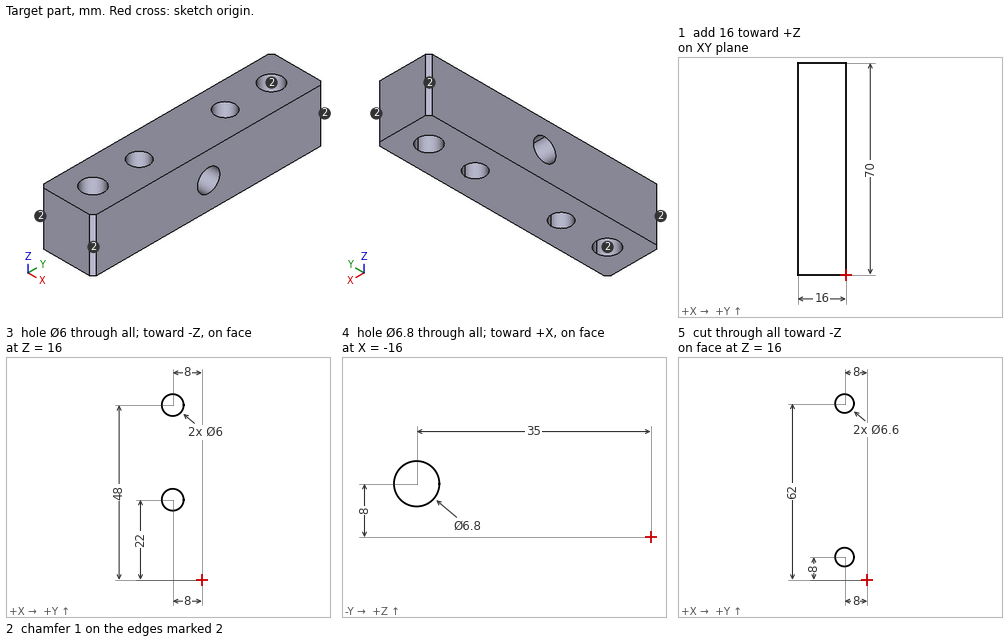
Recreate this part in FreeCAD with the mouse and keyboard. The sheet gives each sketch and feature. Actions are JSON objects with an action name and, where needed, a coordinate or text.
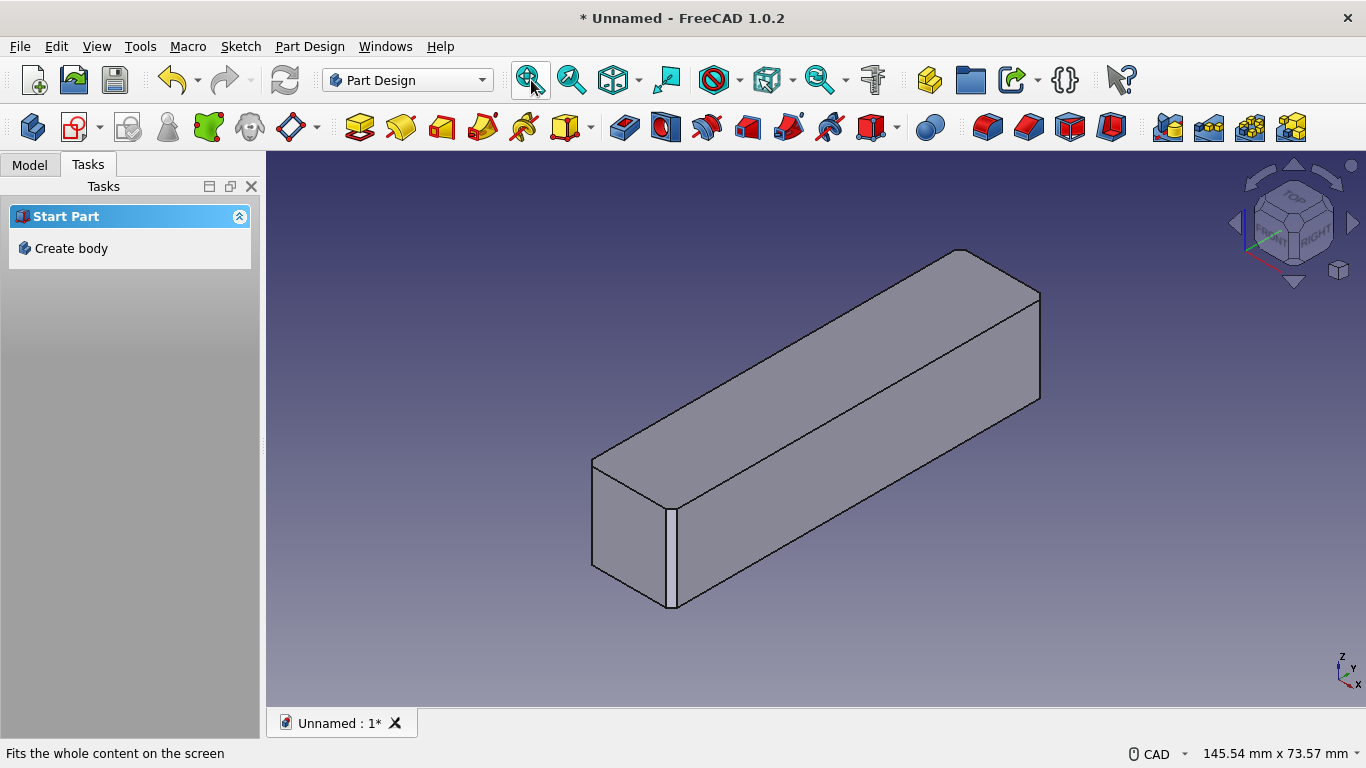
{"action": "left_click", "coordinate": [923, 317]}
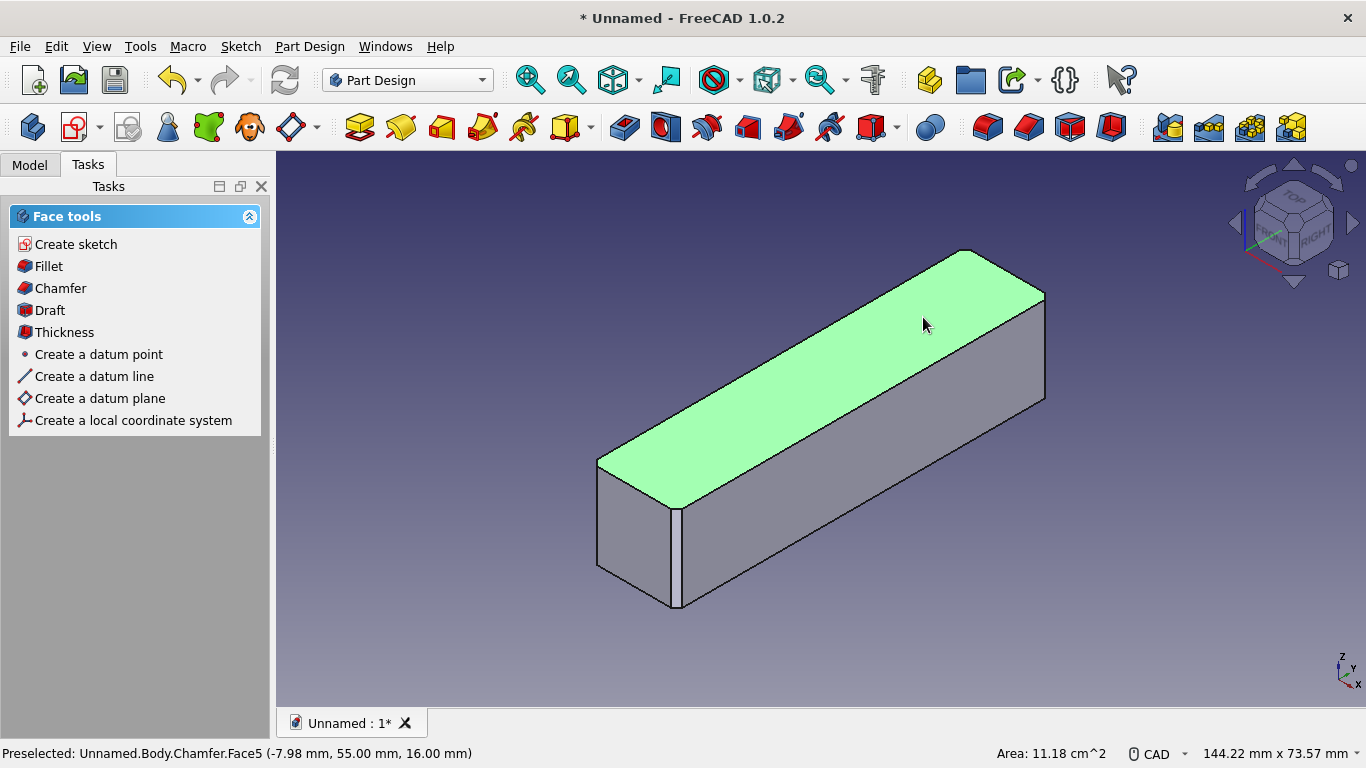
{"action": "left_click", "coordinate": [74, 128]}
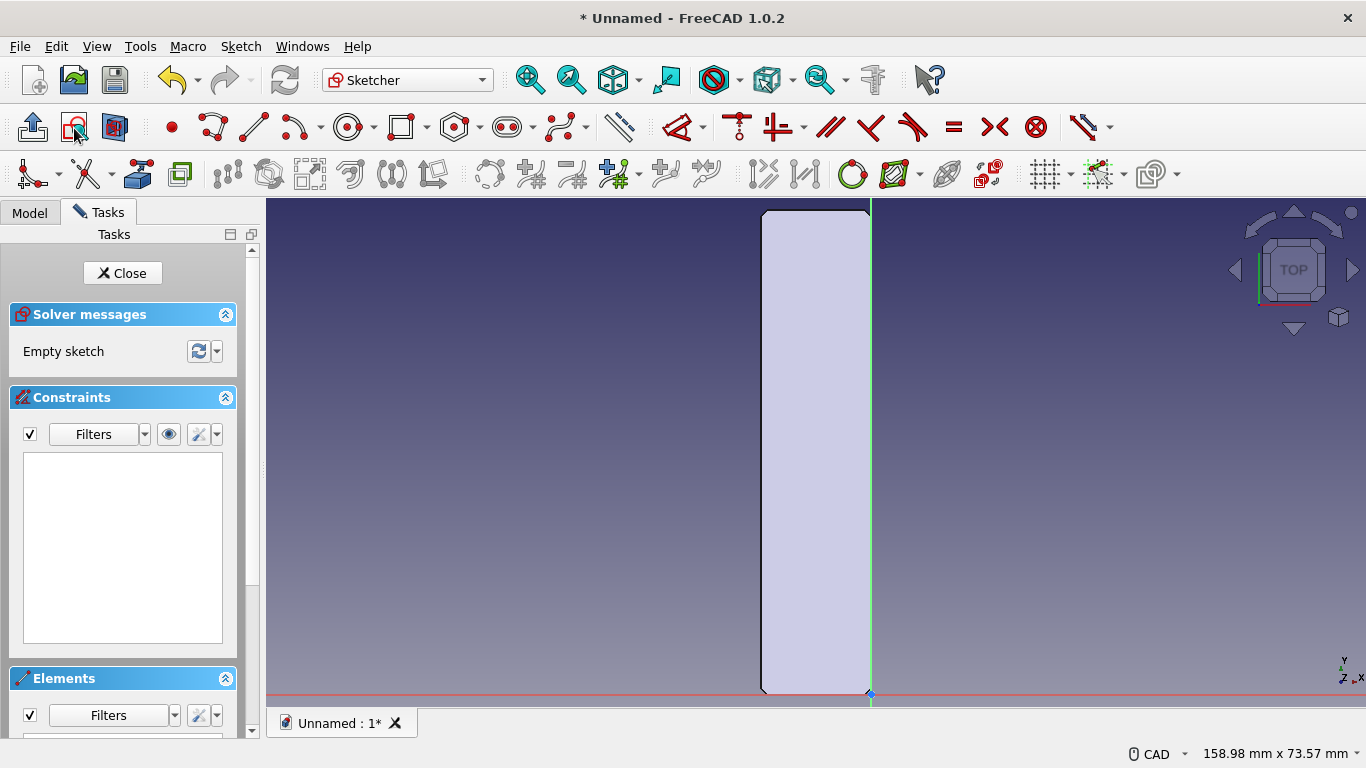
{"action": "scroll", "coordinate": [360, 226], "scroll_direction": "down", "scroll_amount": 1}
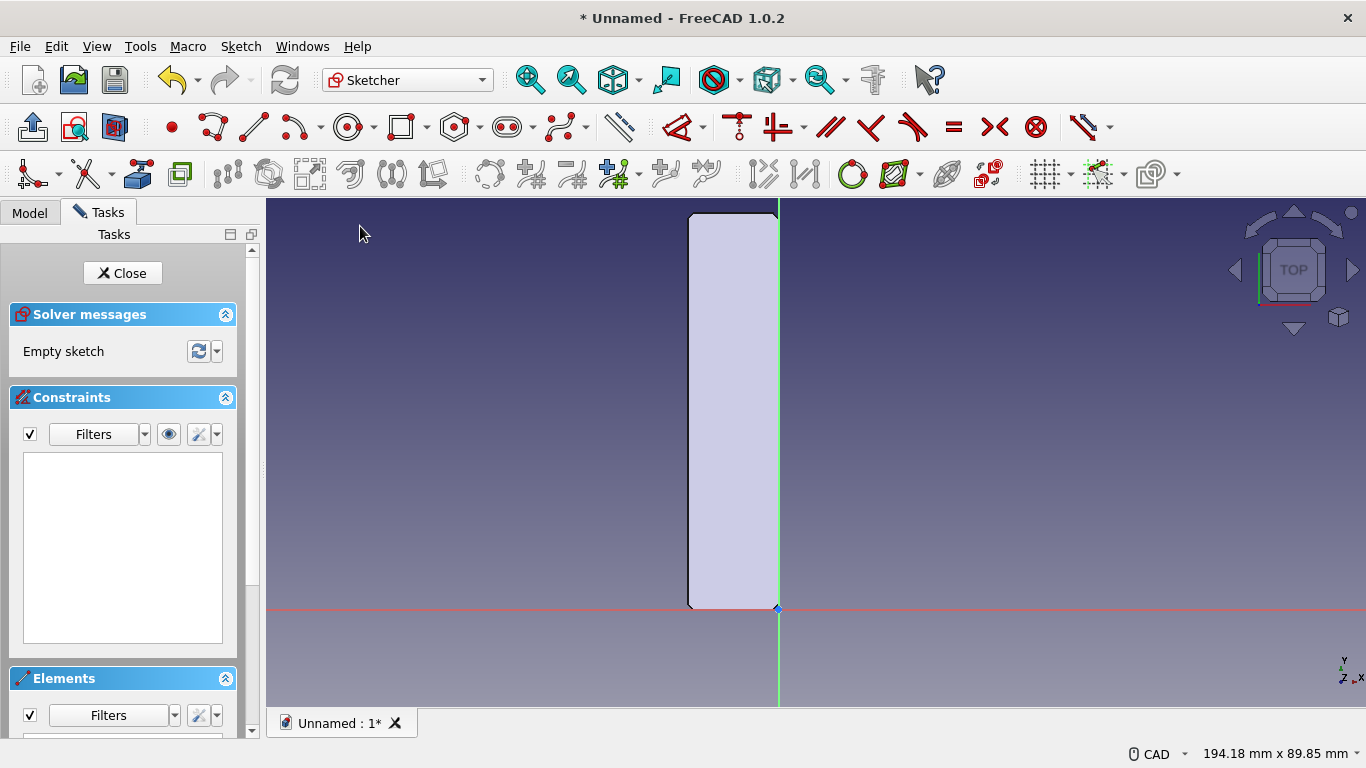
{"action": "left_click", "coordinate": [348, 128]}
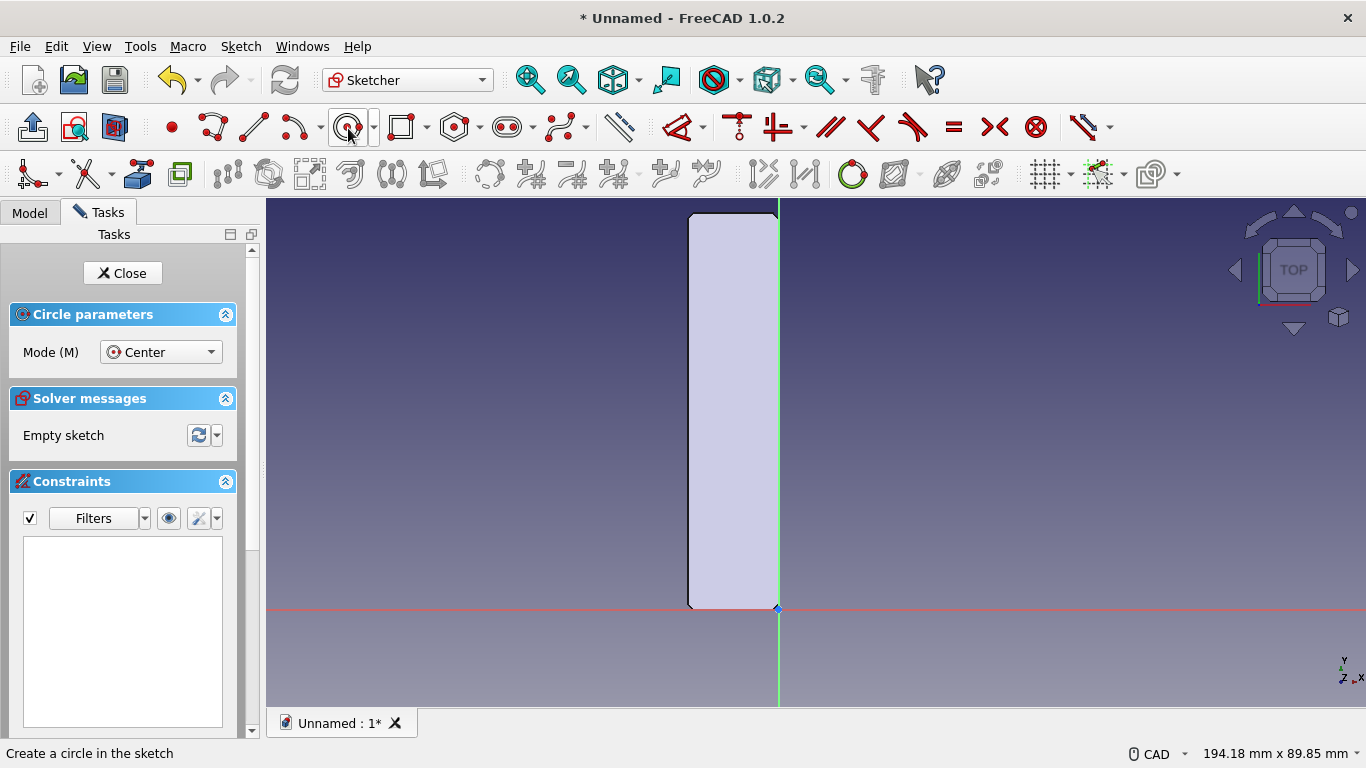
{"action": "scroll", "coordinate": [733, 338], "scroll_direction": "up", "scroll_amount": 2}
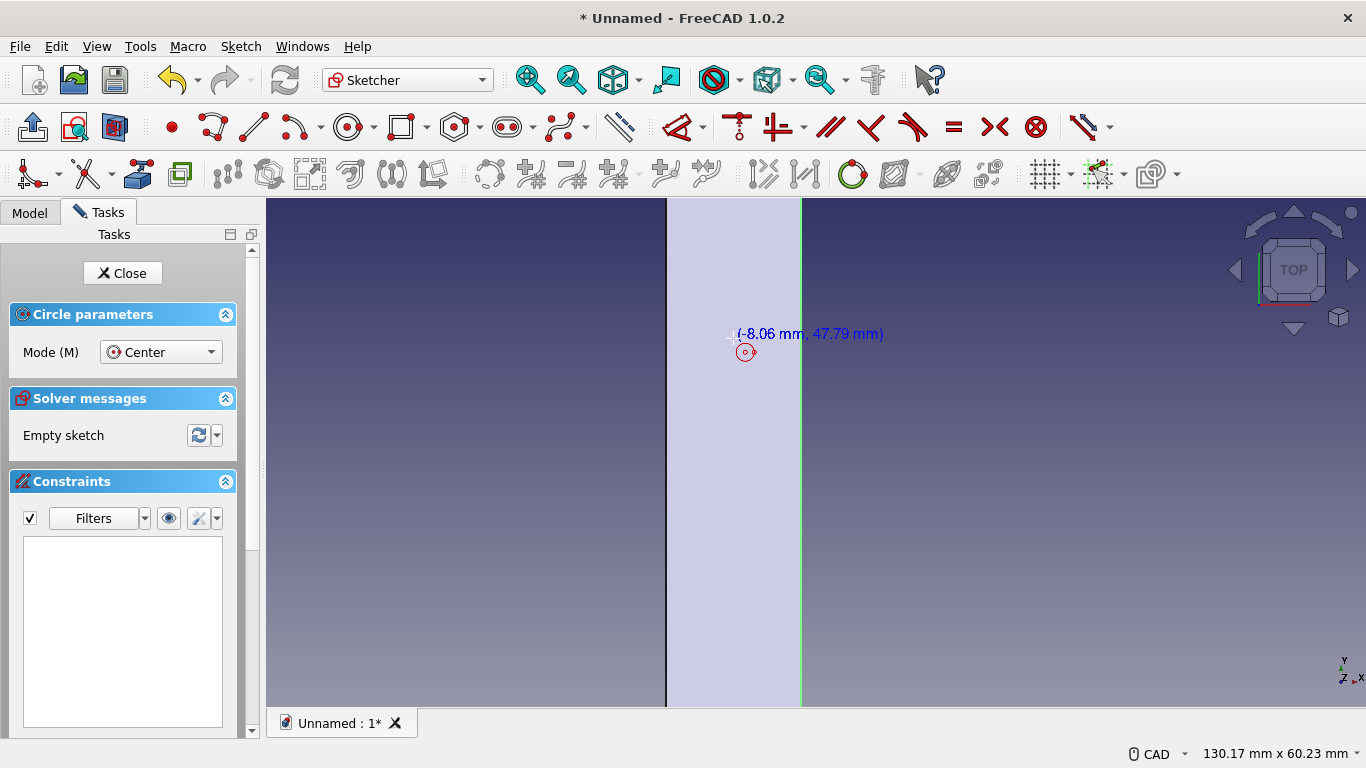
{"action": "left_click", "coordinate": [733, 338]}
{"action": "mouse_move", "coordinate": [751, 320]}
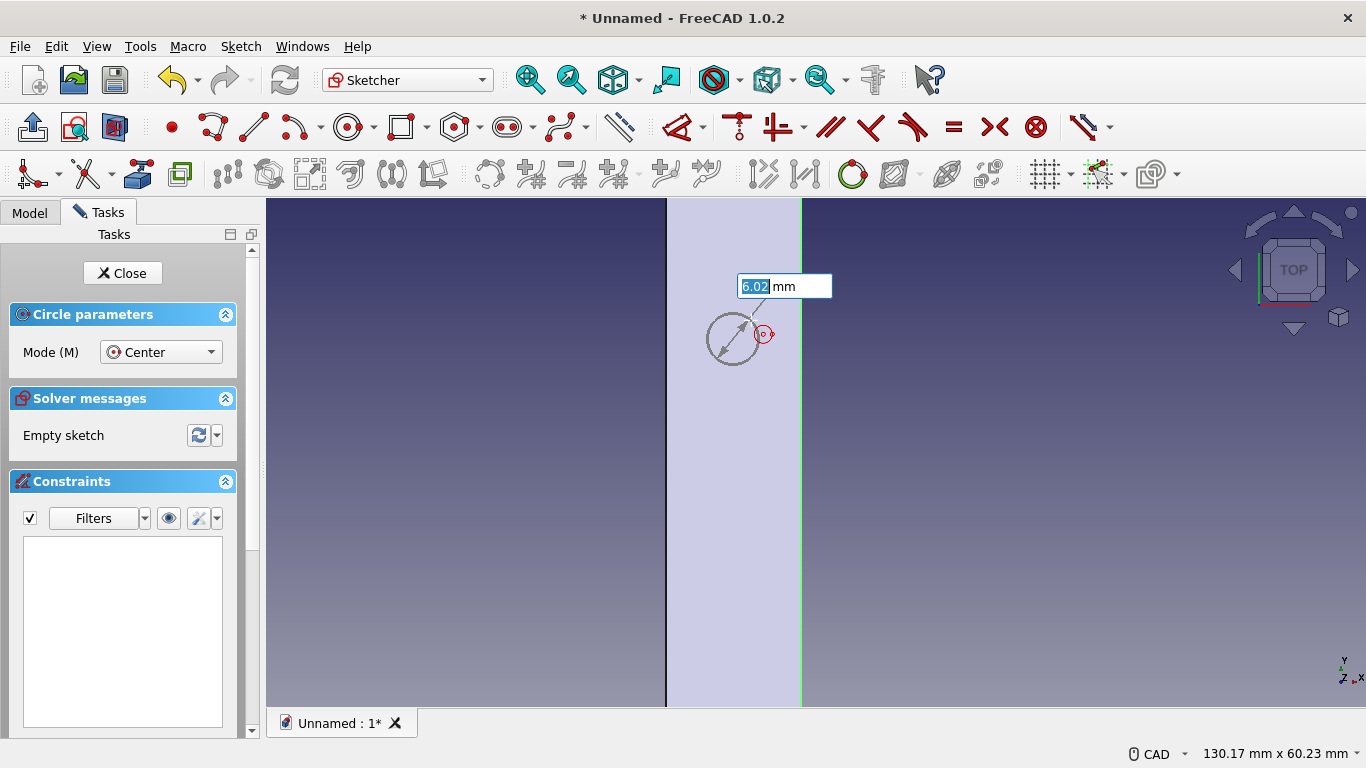
{"action": "type", "text": "6"}
{"action": "key", "text": "Return"}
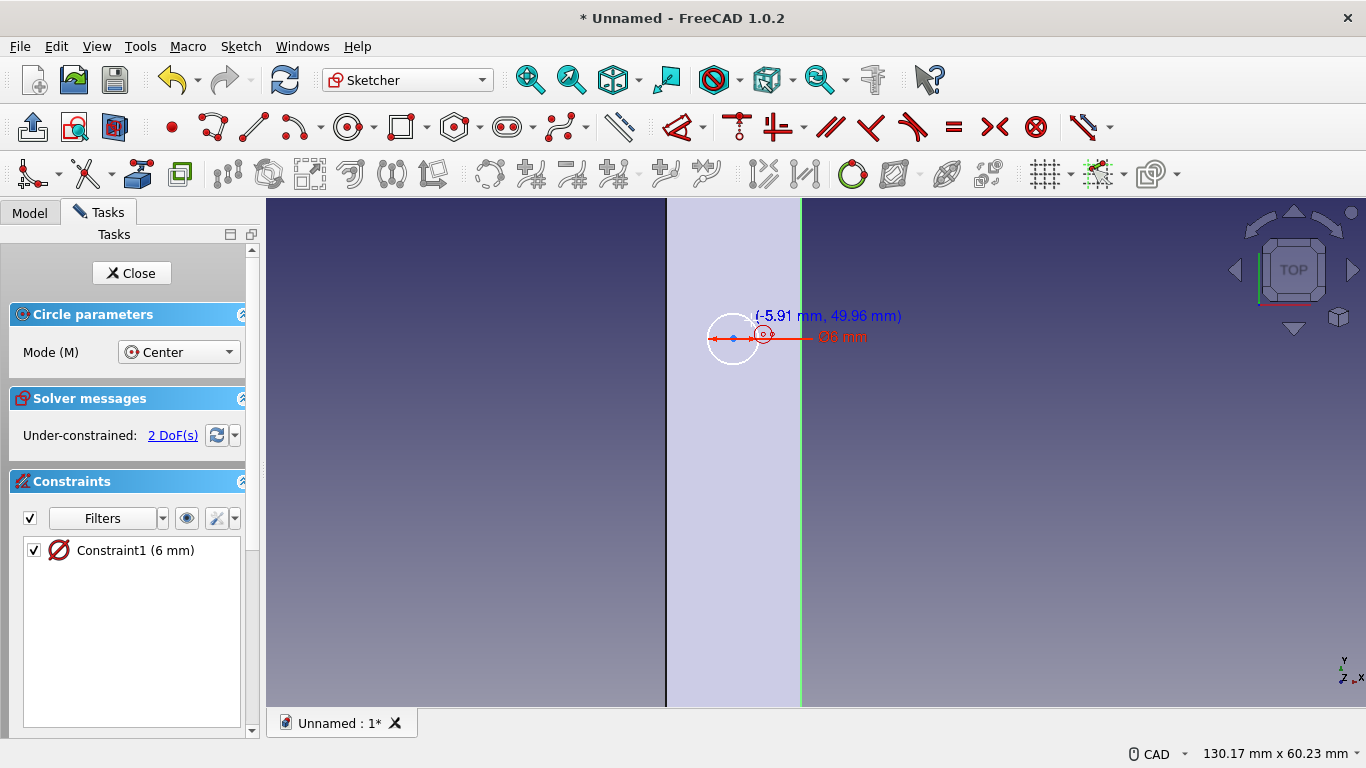
{"action": "left_click", "coordinate": [733, 557]}
{"action": "mouse_move", "coordinate": [751, 539]}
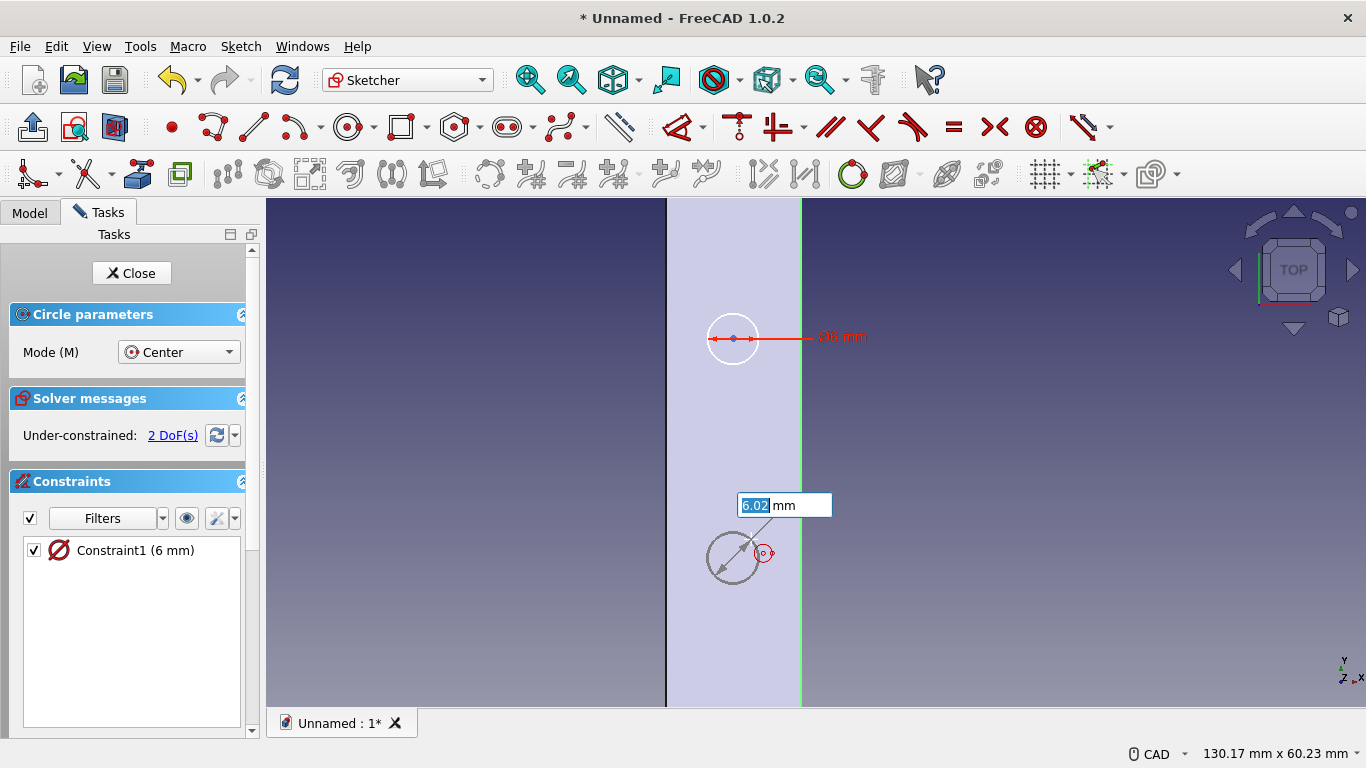
{"action": "type", "text": "6"}
{"action": "key", "text": "Return"}
{"action": "key", "text": "Escape"}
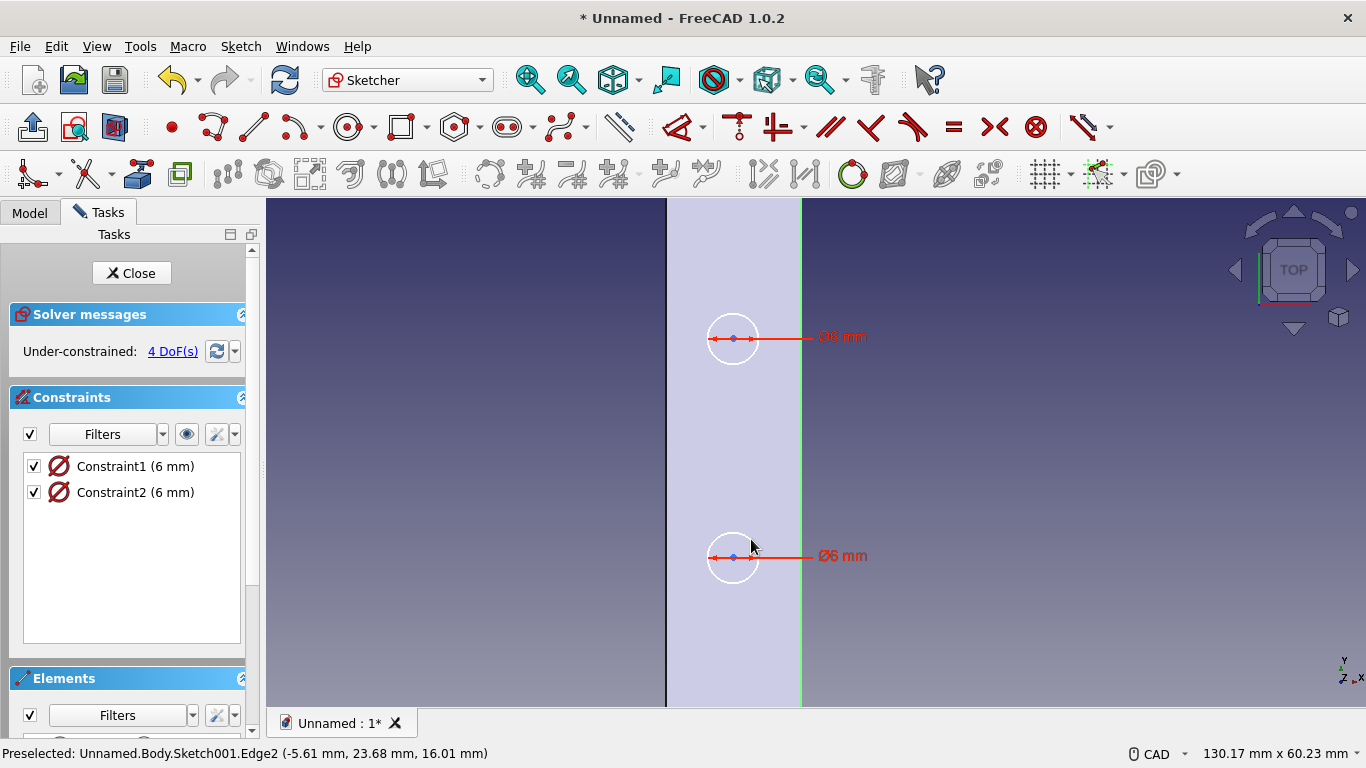
{"action": "left_click", "coordinate": [676, 128]}